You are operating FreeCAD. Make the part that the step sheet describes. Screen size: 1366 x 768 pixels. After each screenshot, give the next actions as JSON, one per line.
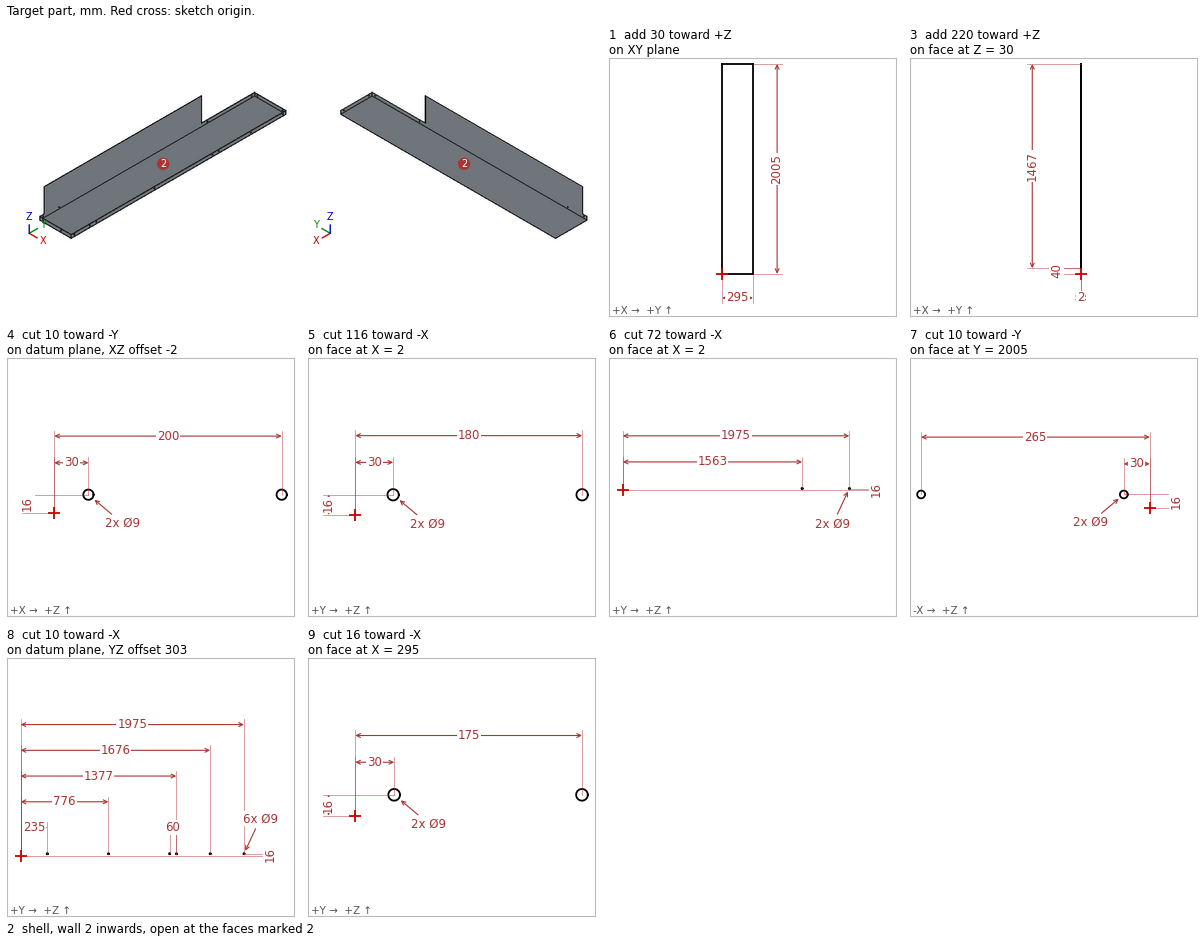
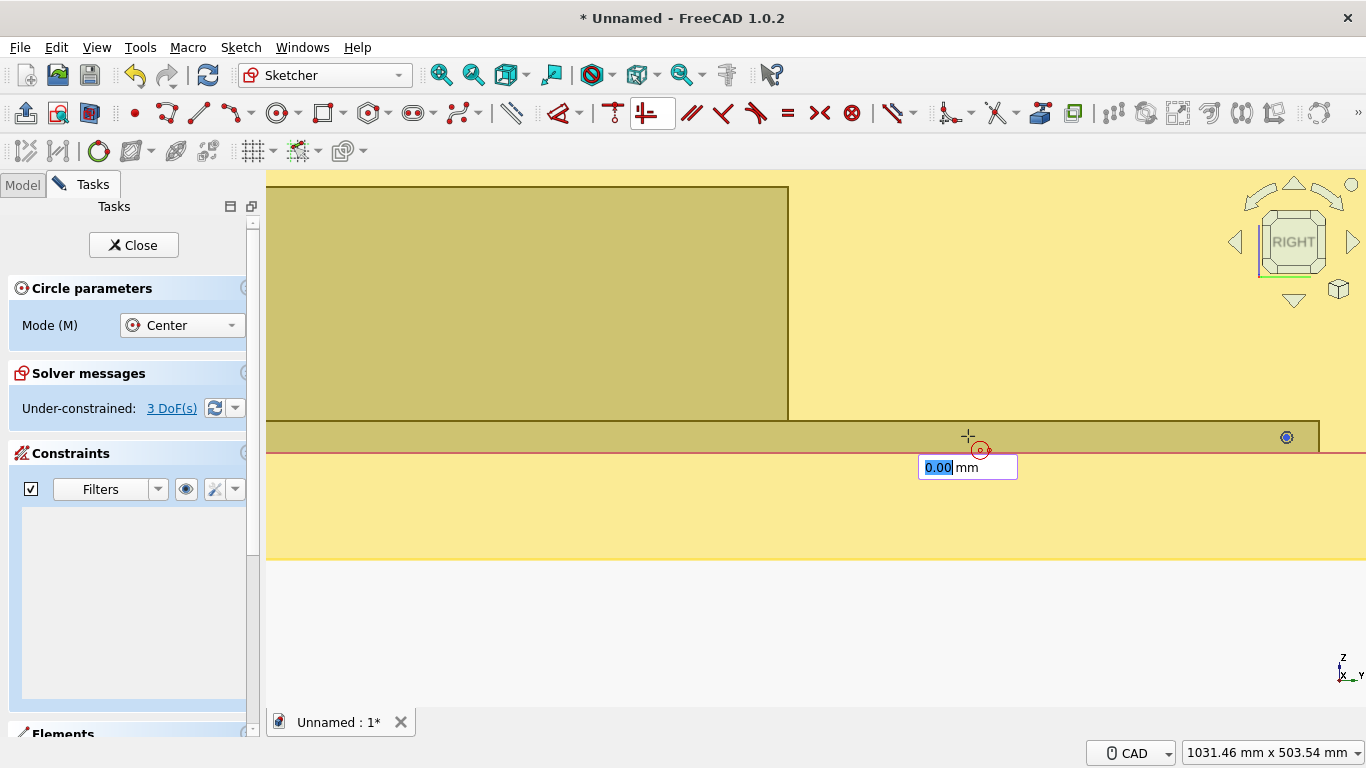
{"action": "scroll", "coordinate": [972, 433], "scroll_direction": "up", "scroll_amount": 6}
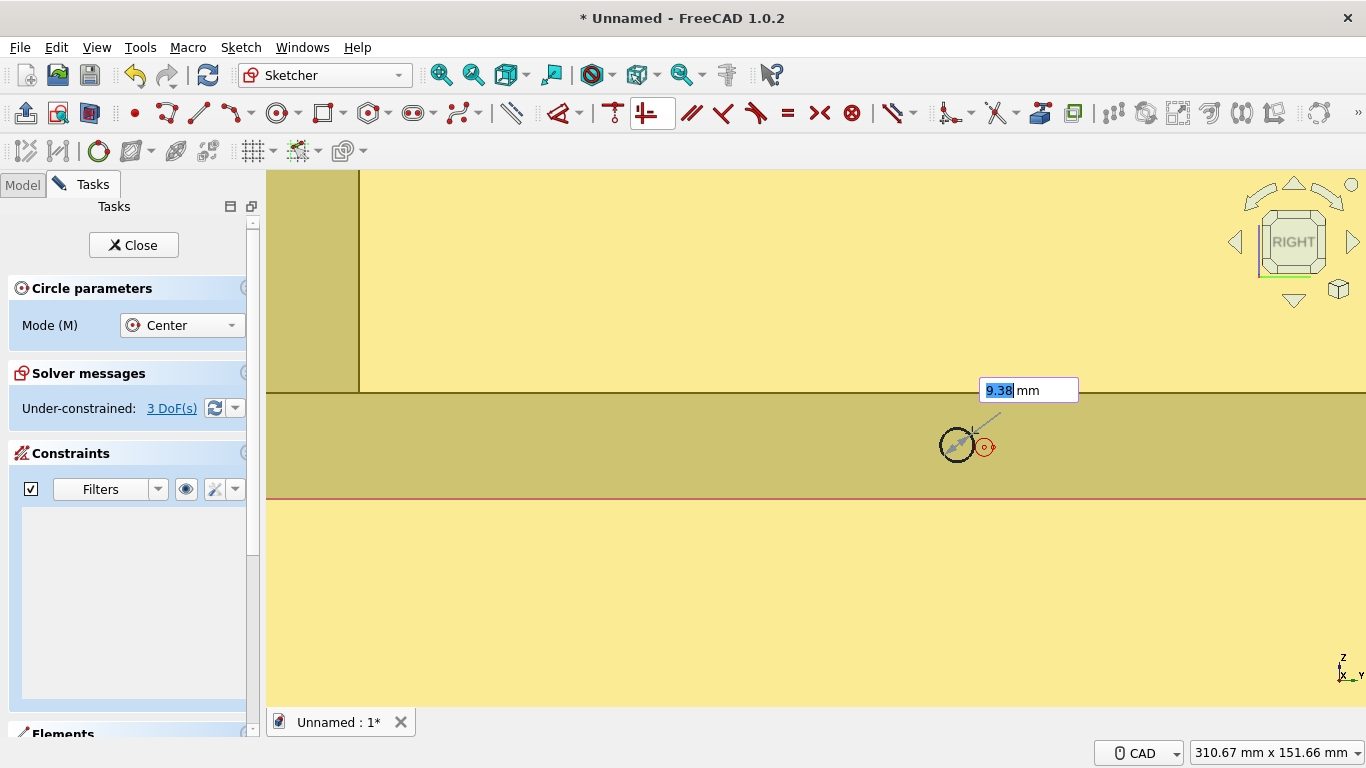
{"action": "left_click", "coordinate": [969, 431]}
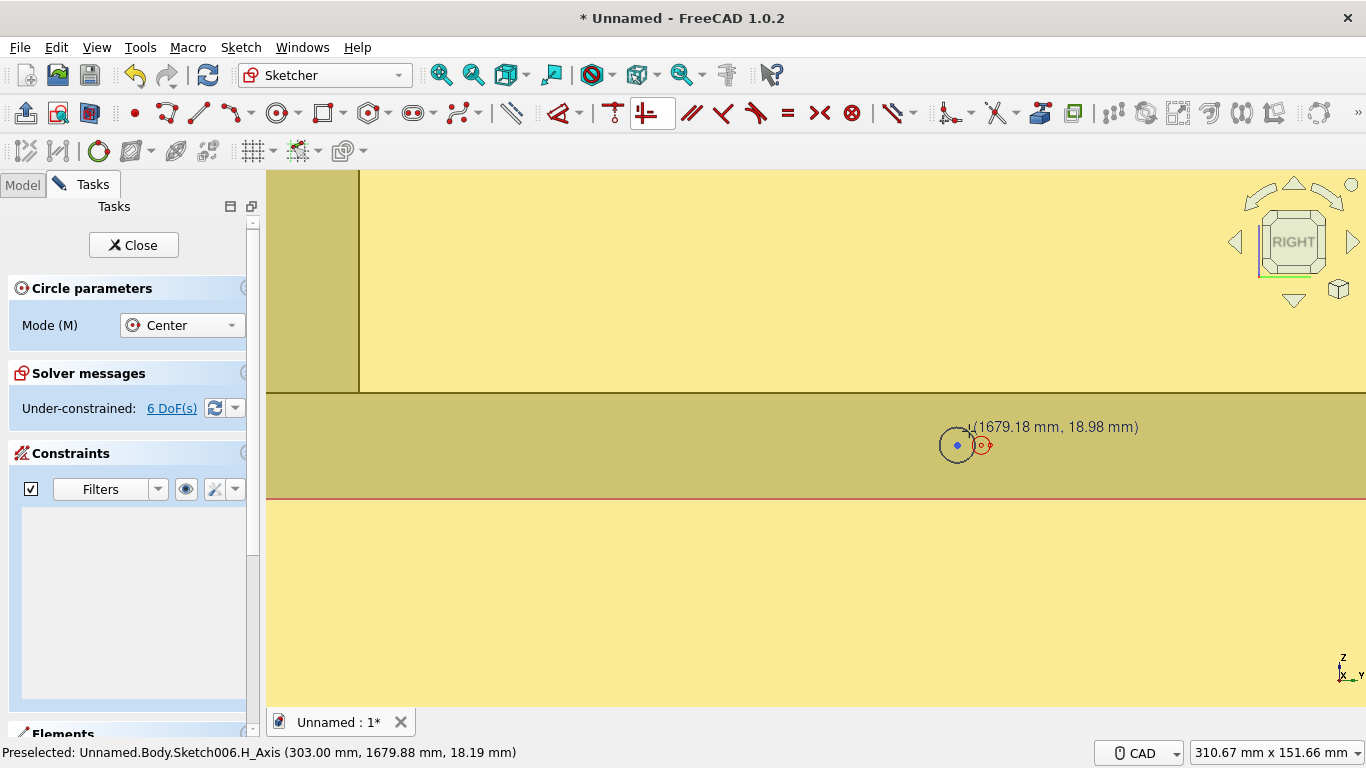
{"action": "scroll", "coordinate": [969, 436], "scroll_direction": "down", "scroll_amount": 12}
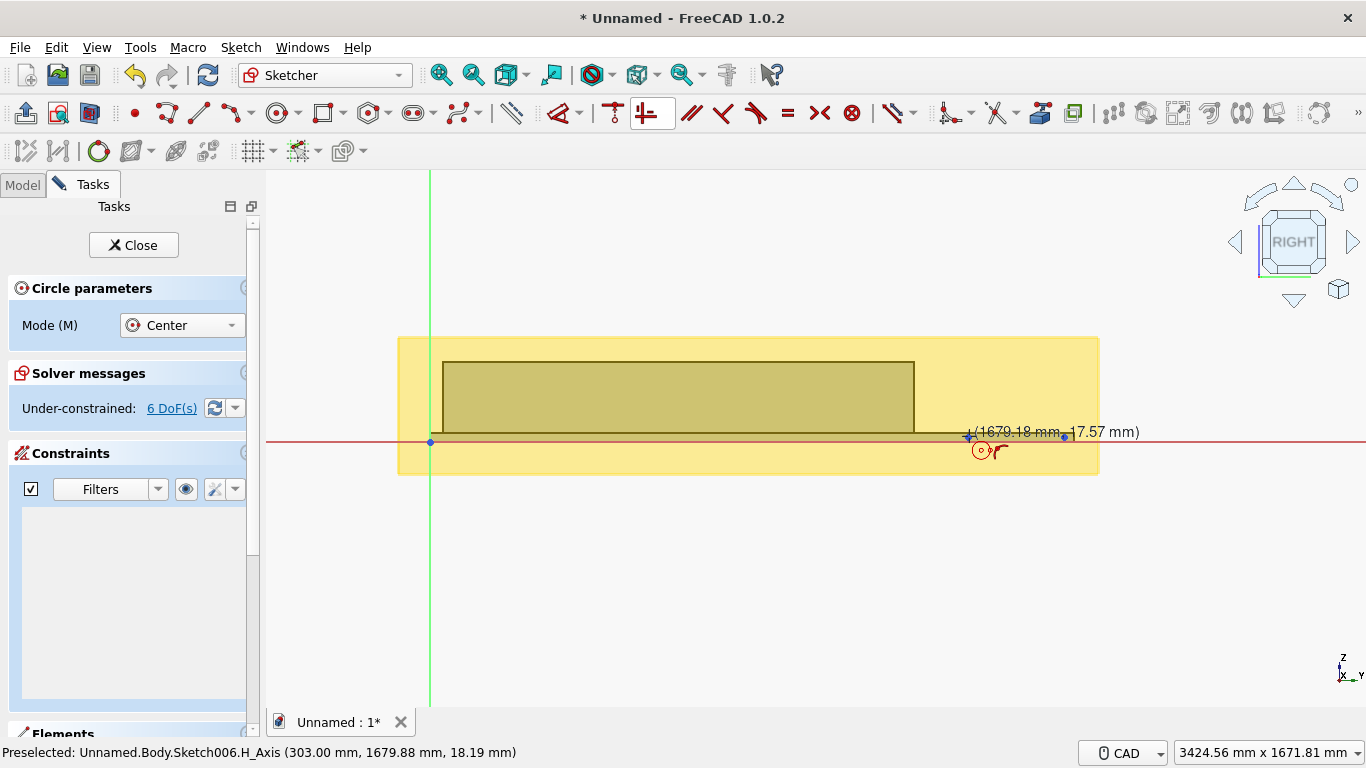
{"action": "scroll", "coordinate": [873, 437], "scroll_direction": "up", "scroll_amount": 14}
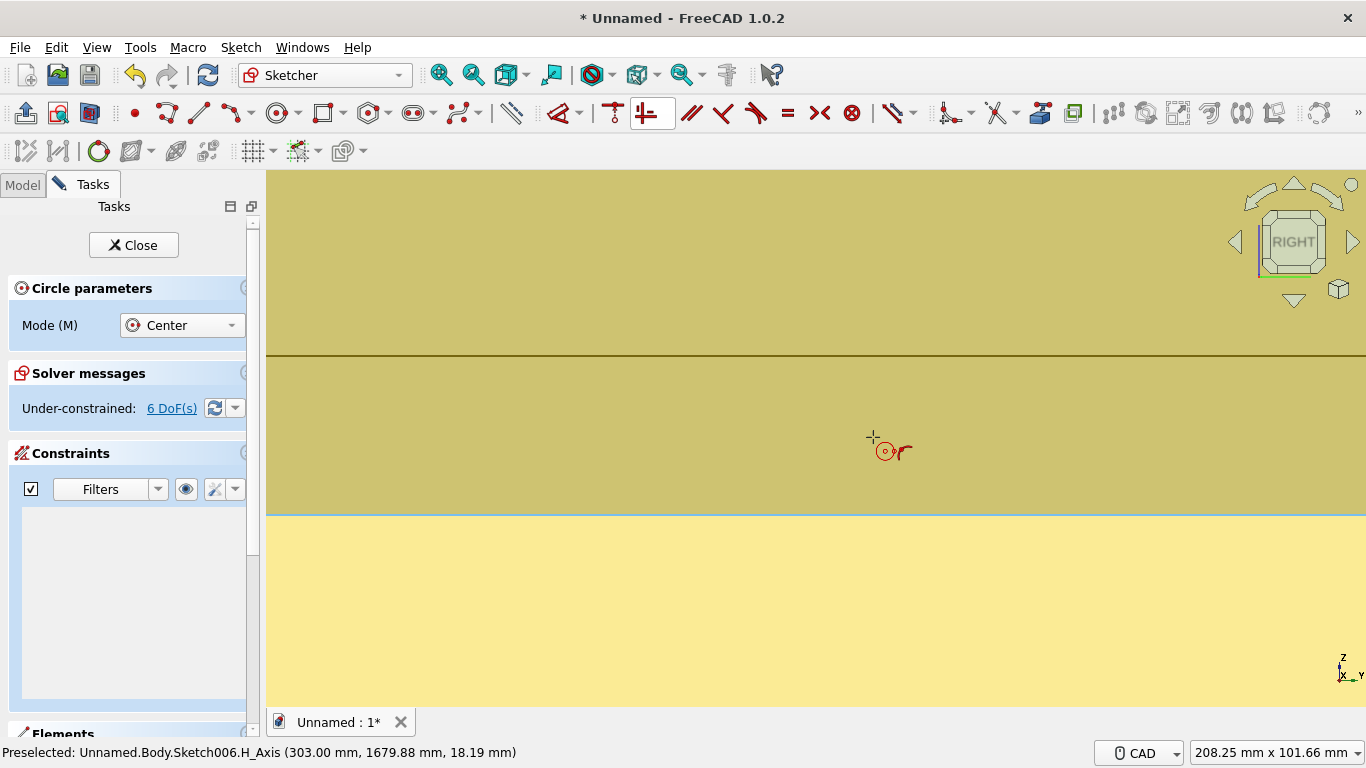
{"action": "scroll", "coordinate": [873, 437], "scroll_direction": "down", "scroll_amount": 14}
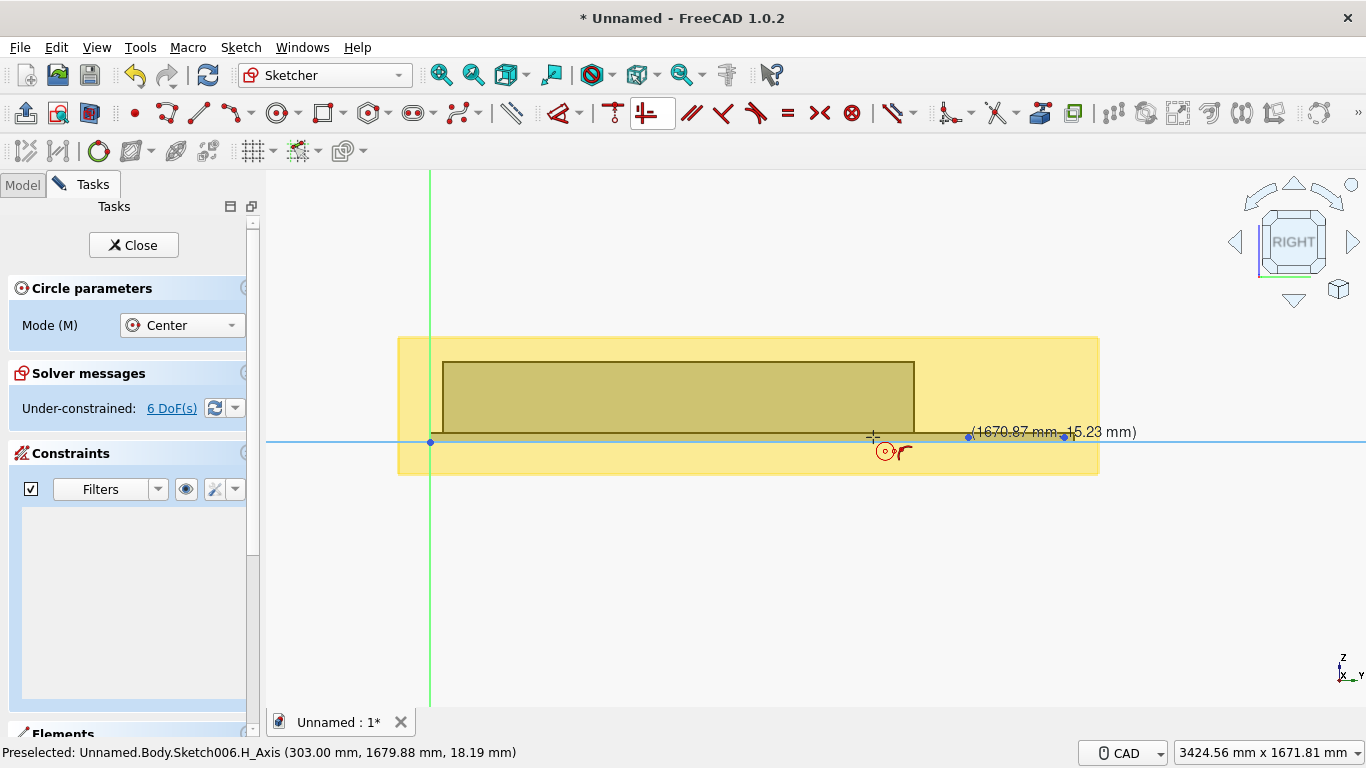
{"action": "scroll", "coordinate": [873, 437], "scroll_direction": "up", "scroll_amount": 6}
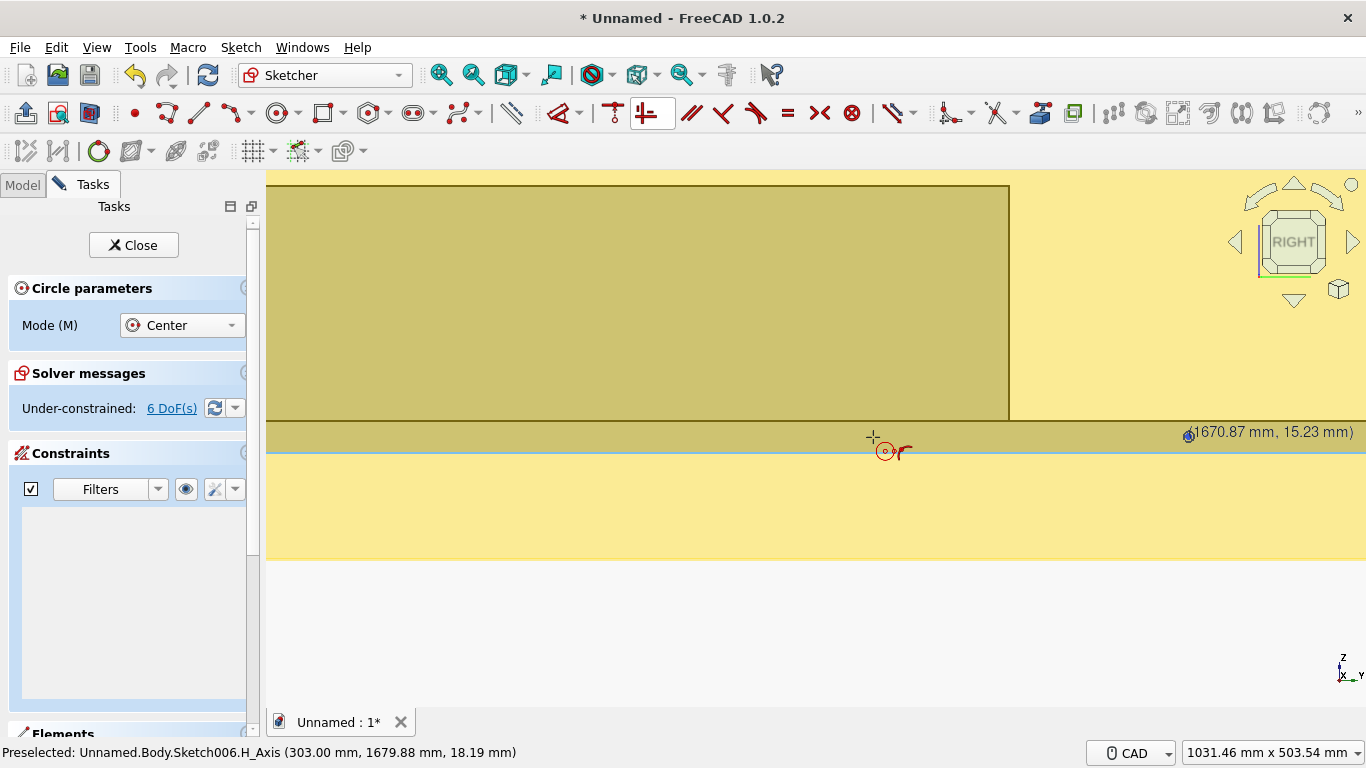
{"action": "left_click", "coordinate": [870, 436]}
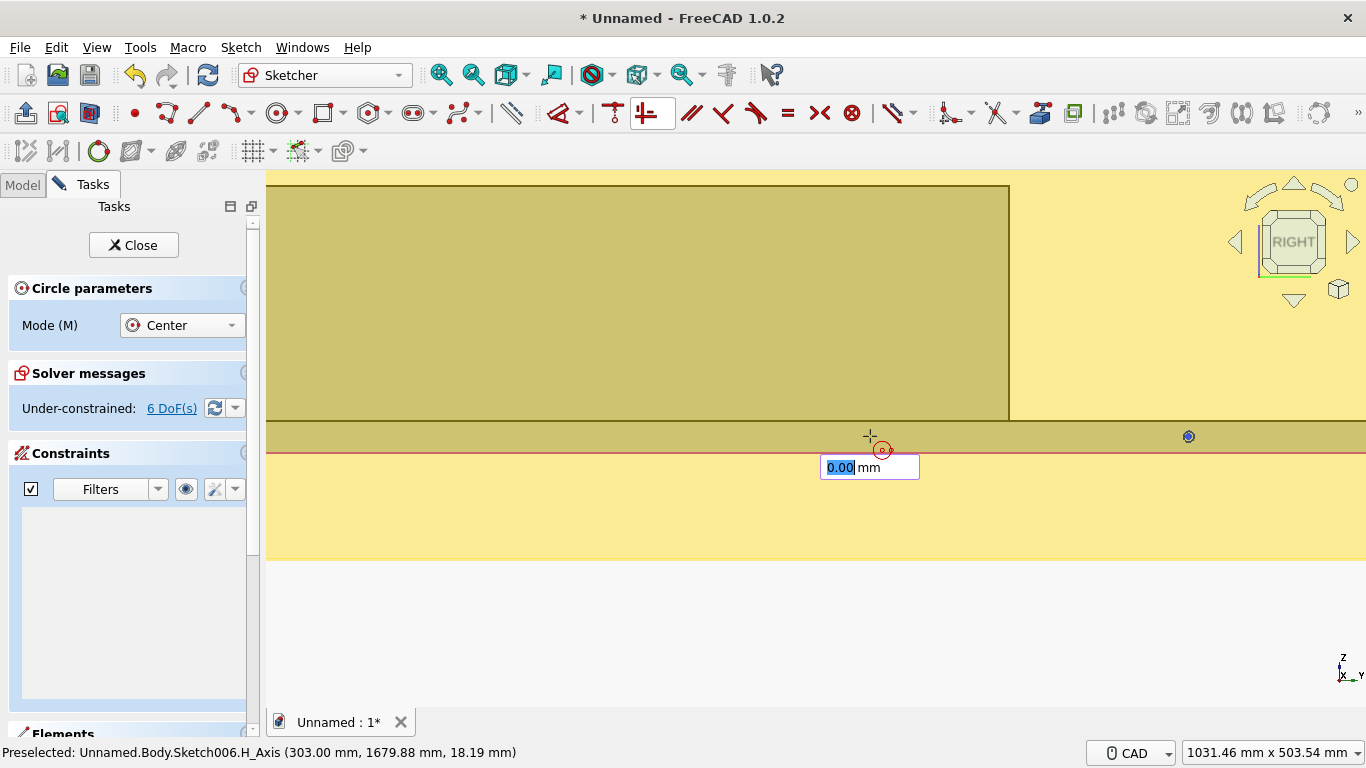
{"action": "scroll", "coordinate": [874, 433], "scroll_direction": "up", "scroll_amount": 6}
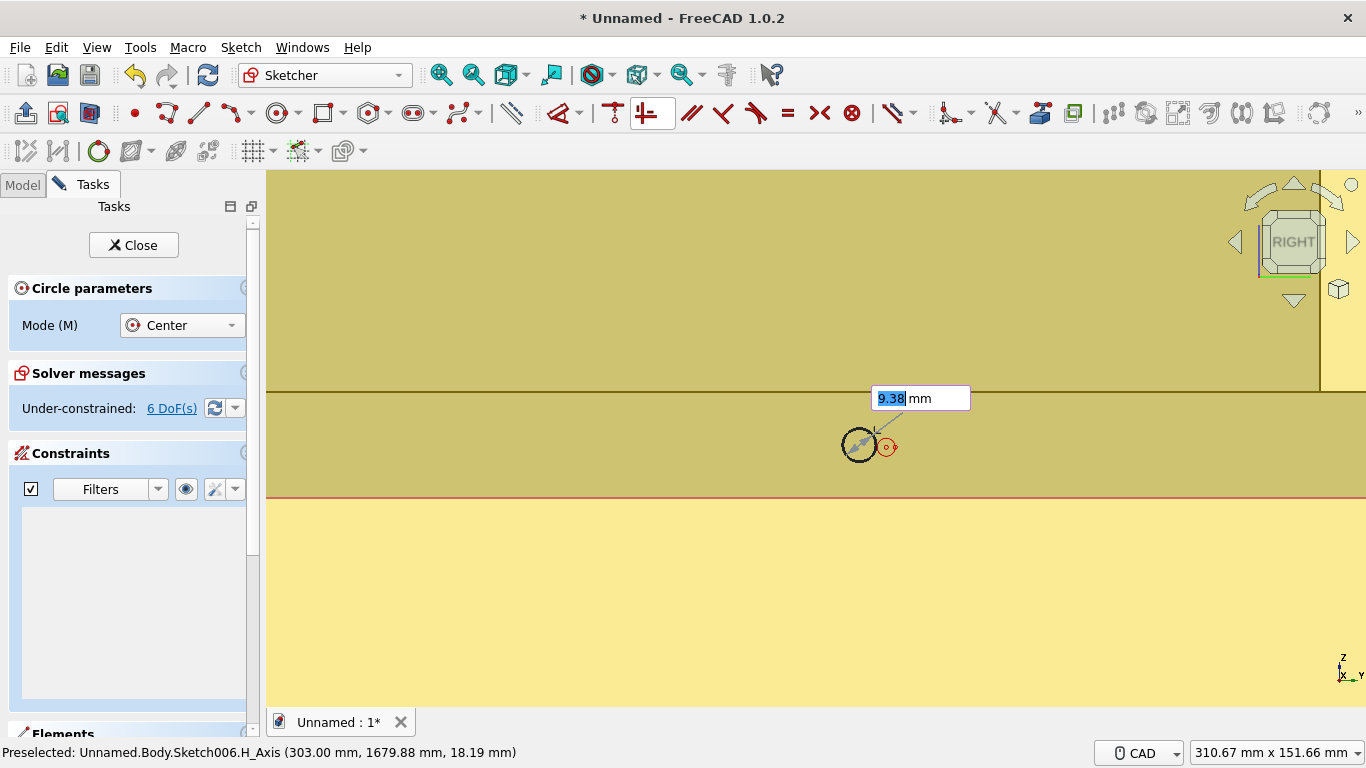
{"action": "left_click", "coordinate": [871, 431]}